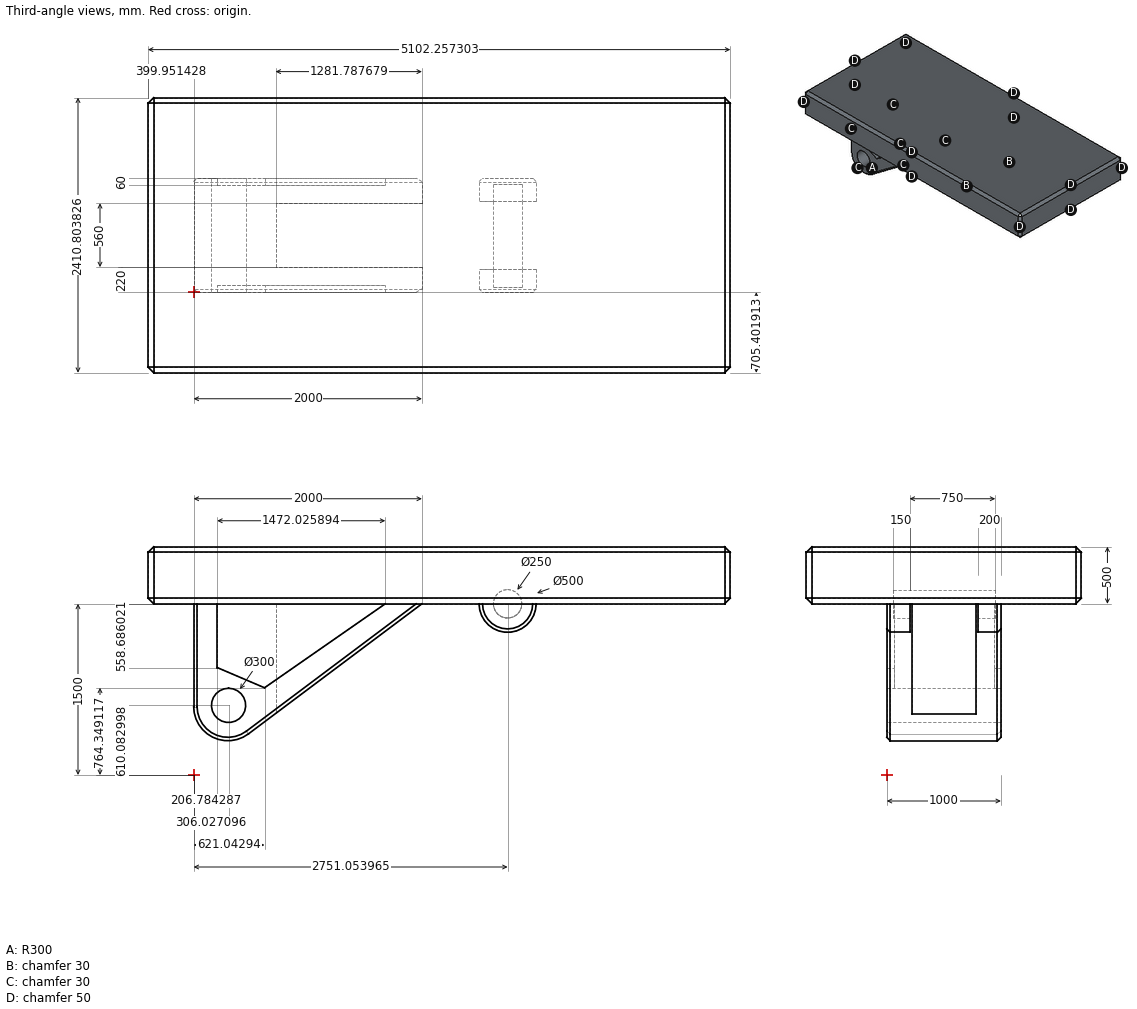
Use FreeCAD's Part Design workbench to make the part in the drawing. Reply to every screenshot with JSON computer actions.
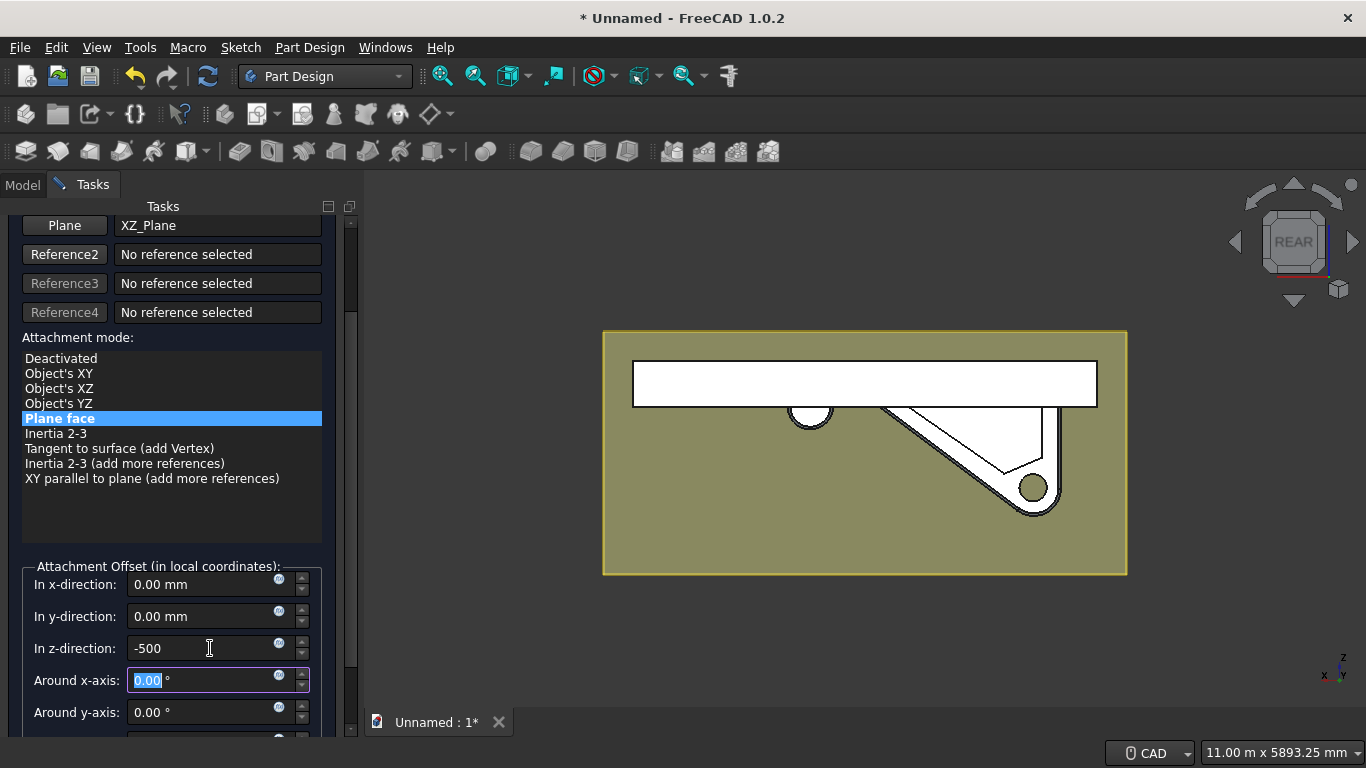
{"action": "scroll", "coordinate": [351, 476], "scroll_direction": "up", "scroll_amount": 3}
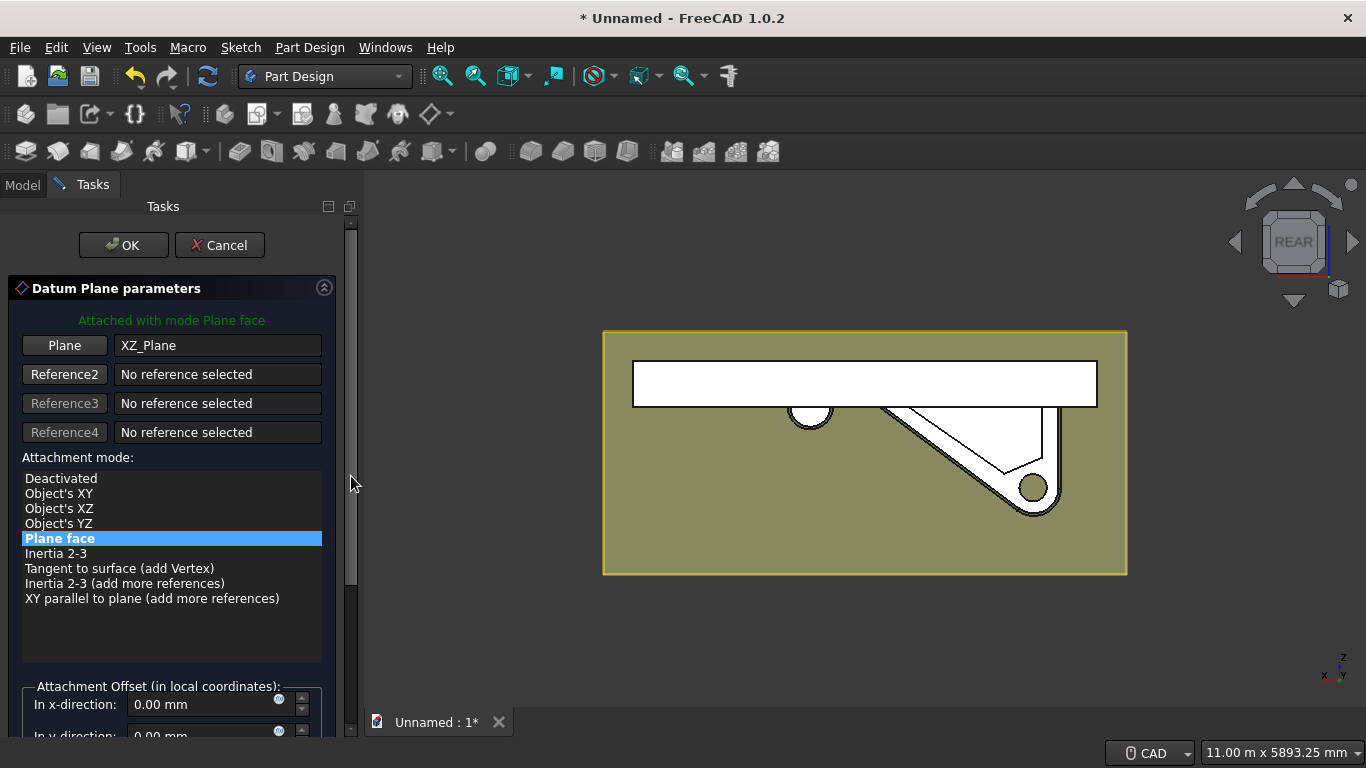
{"action": "left_click", "coordinate": [124, 245]}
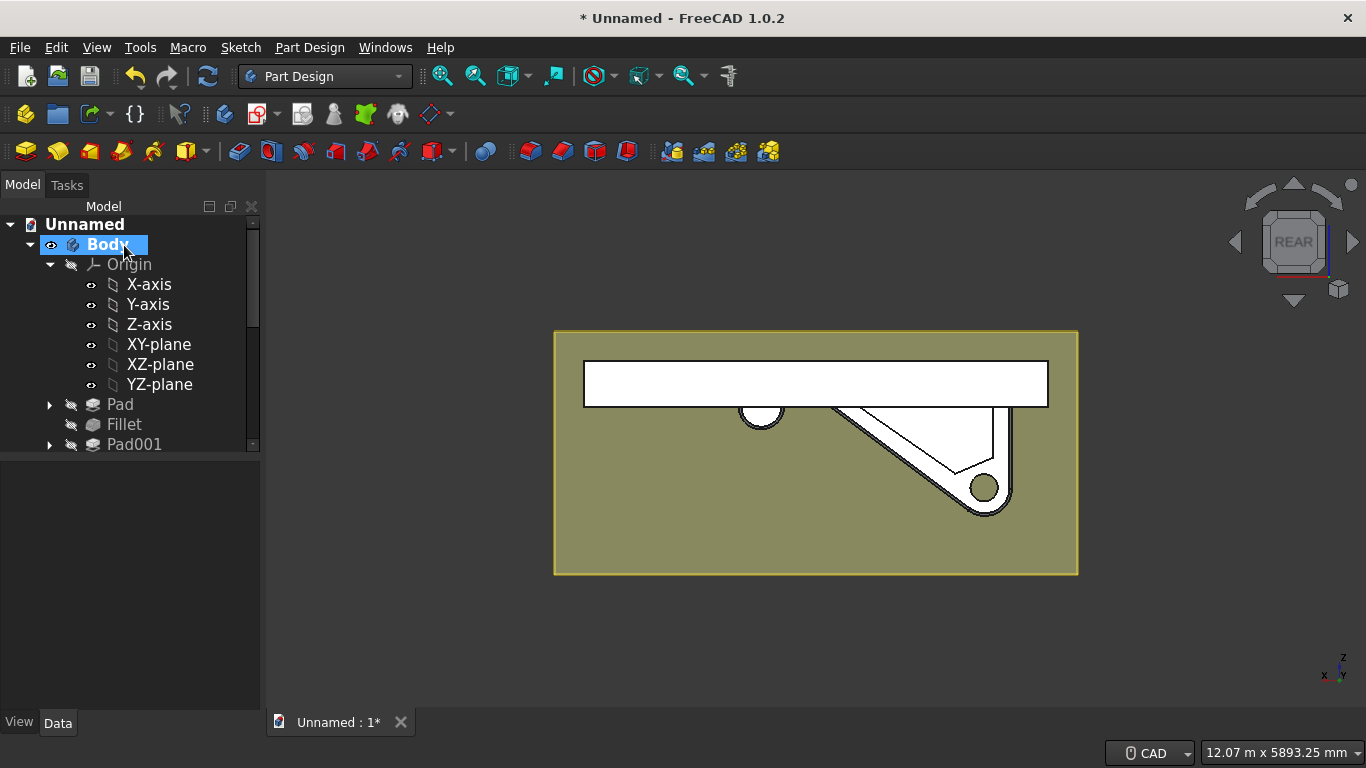
{"action": "scroll", "coordinate": [100, 340], "scroll_direction": "down", "scroll_amount": 3}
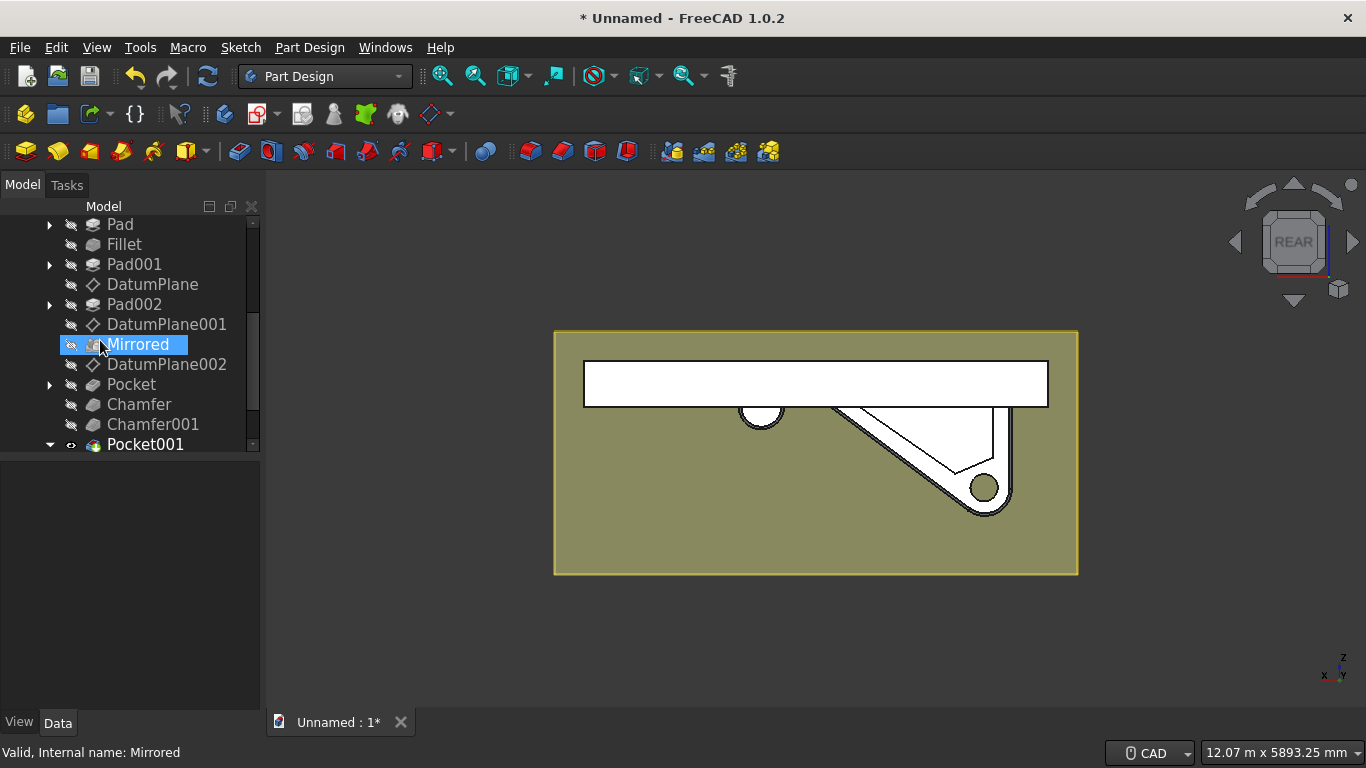
{"action": "left_click", "coordinate": [116, 445]}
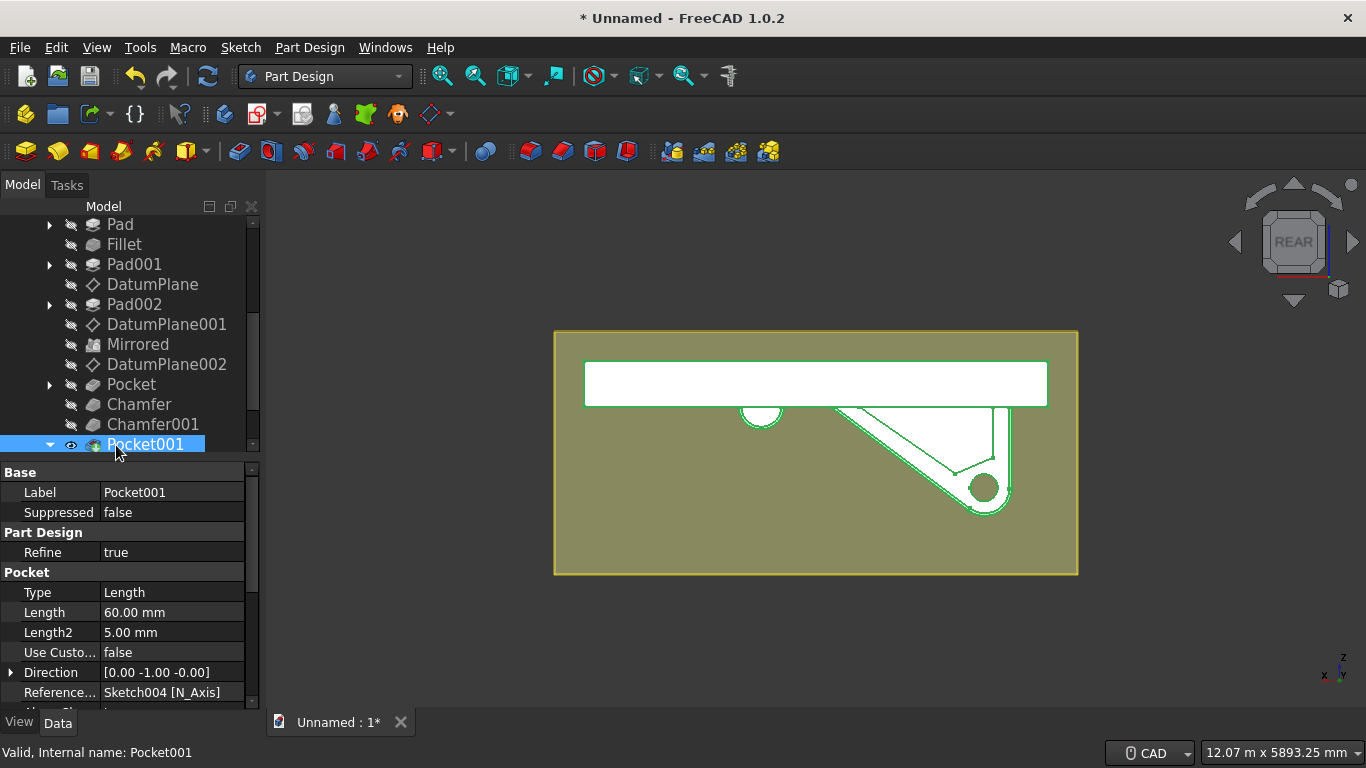
{"action": "left_click", "coordinate": [672, 152]}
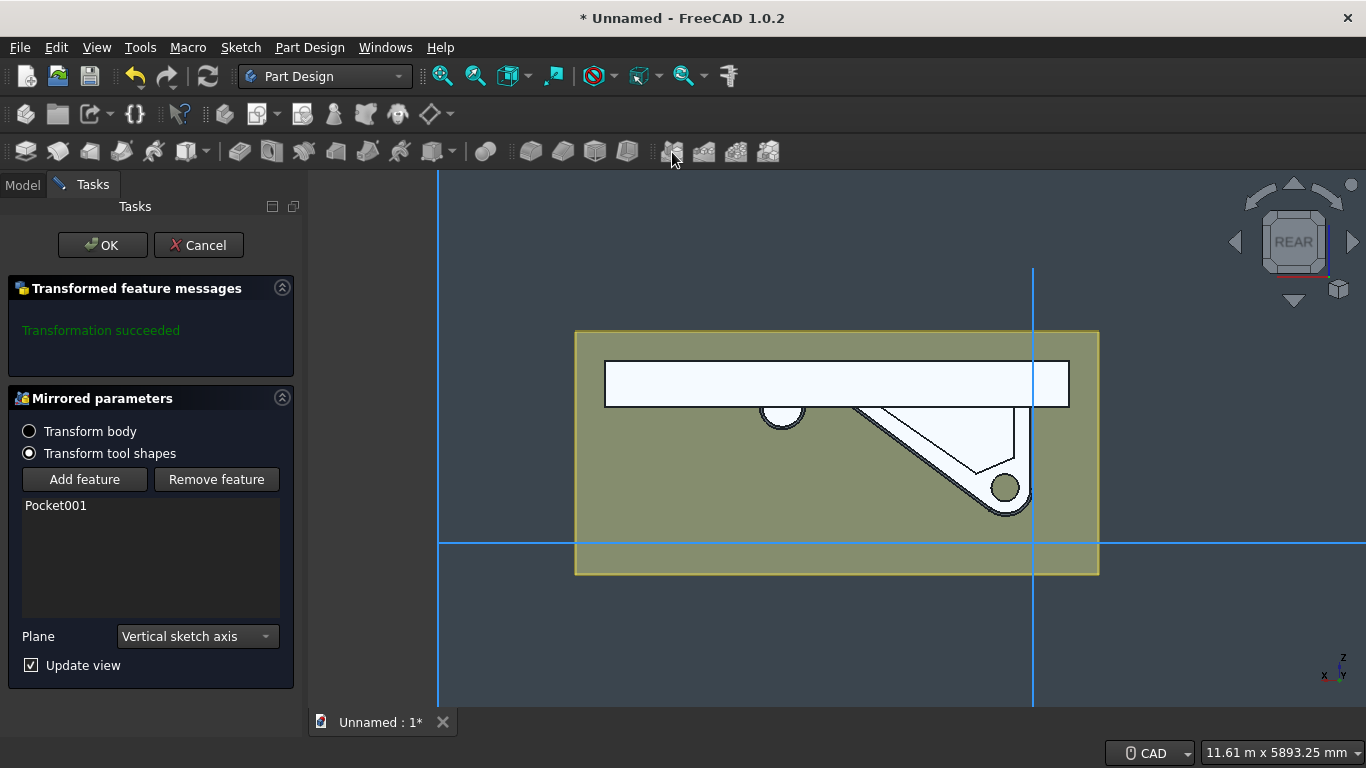
{"action": "left_click", "coordinate": [198, 636]}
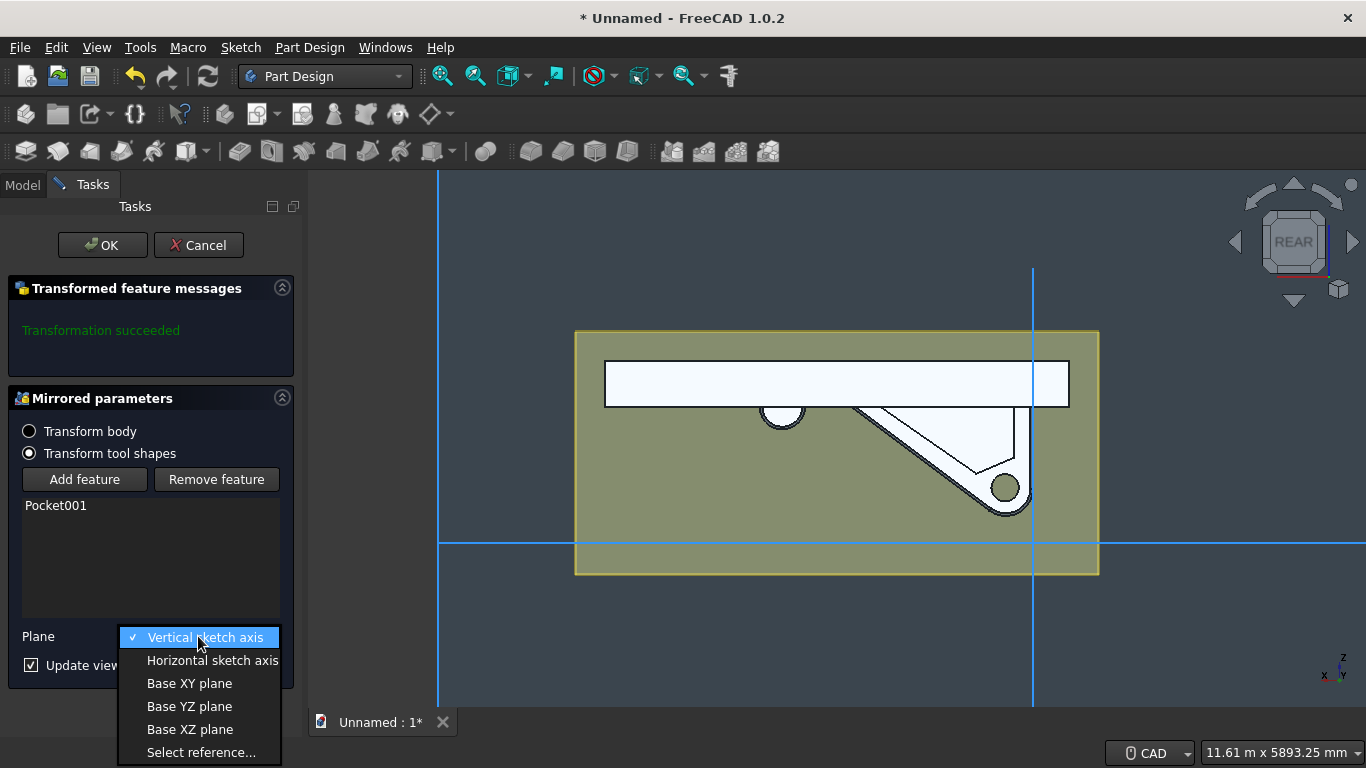
{"action": "left_click", "coordinate": [198, 752]}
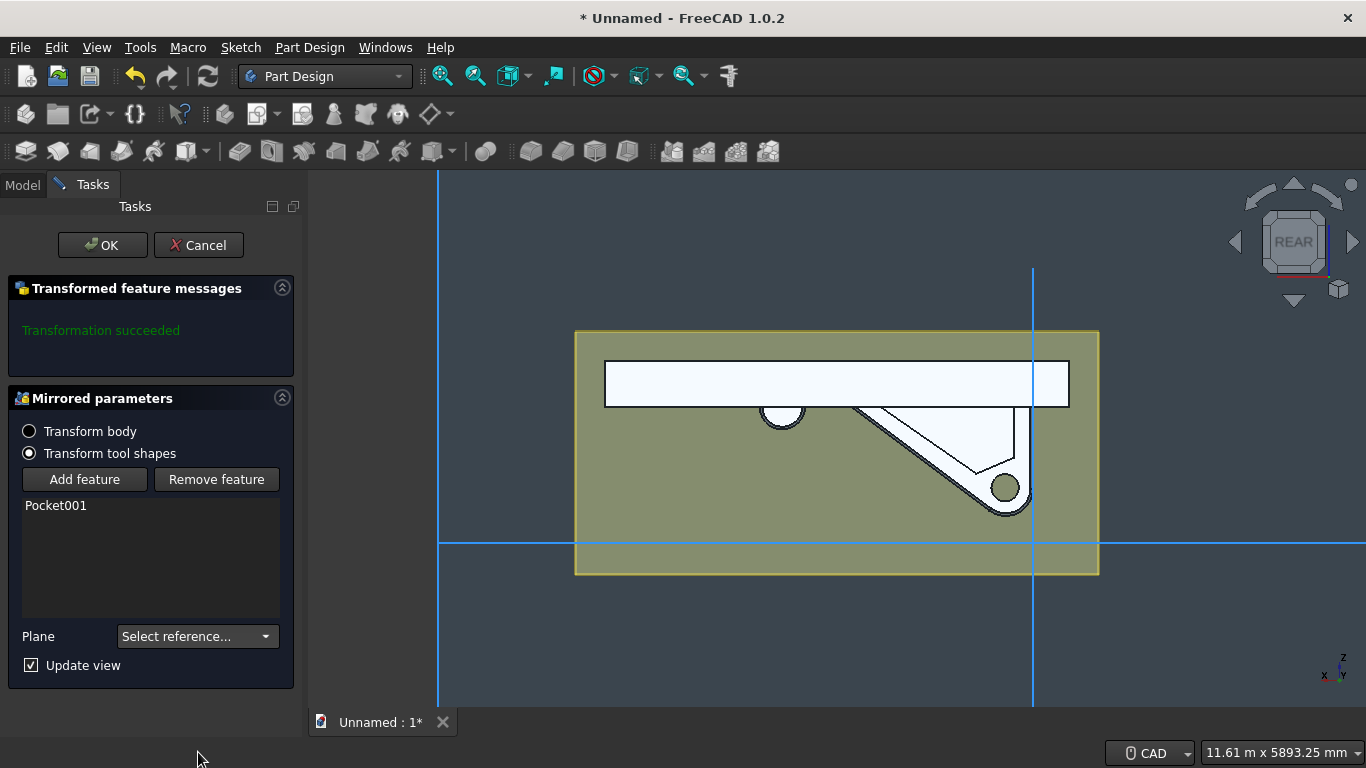
{"action": "left_click", "coordinate": [23, 184]}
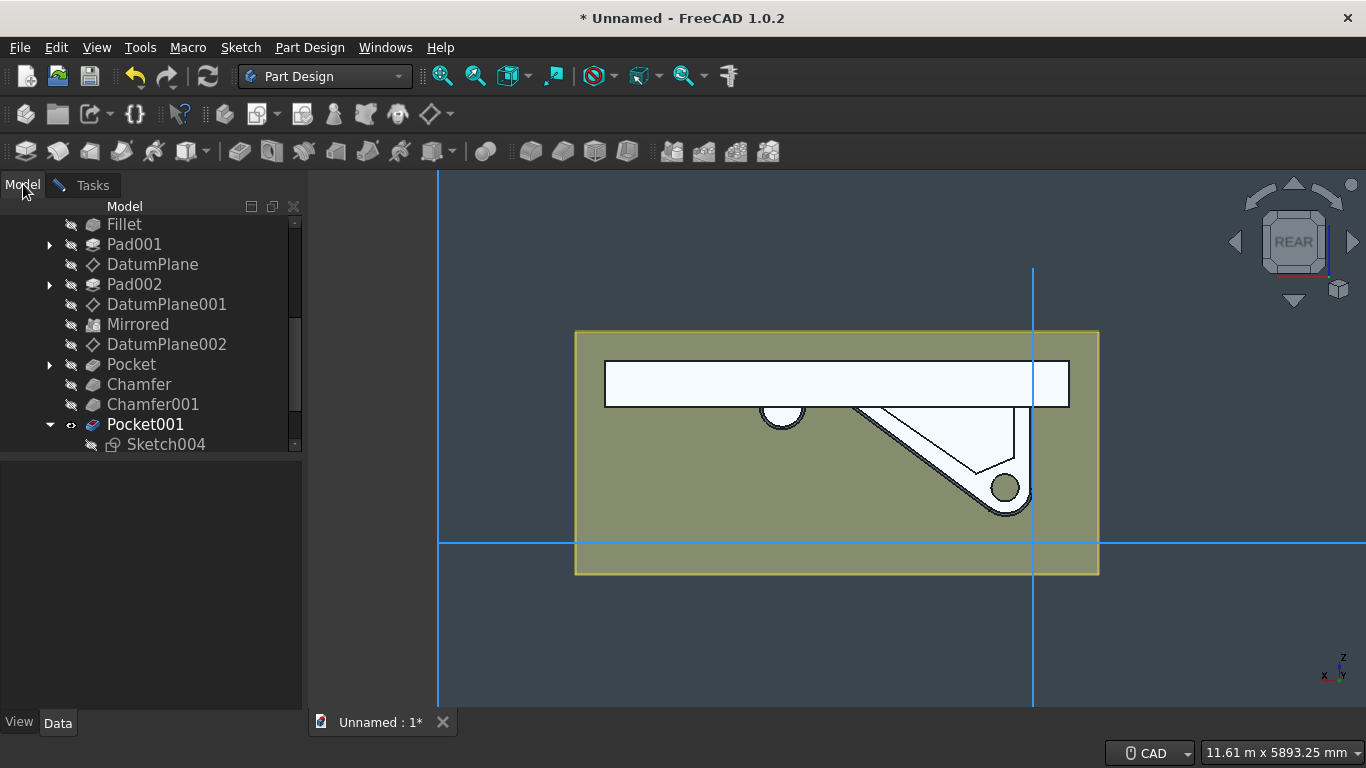
{"action": "scroll", "coordinate": [140, 340], "scroll_direction": "down", "scroll_amount": 3}